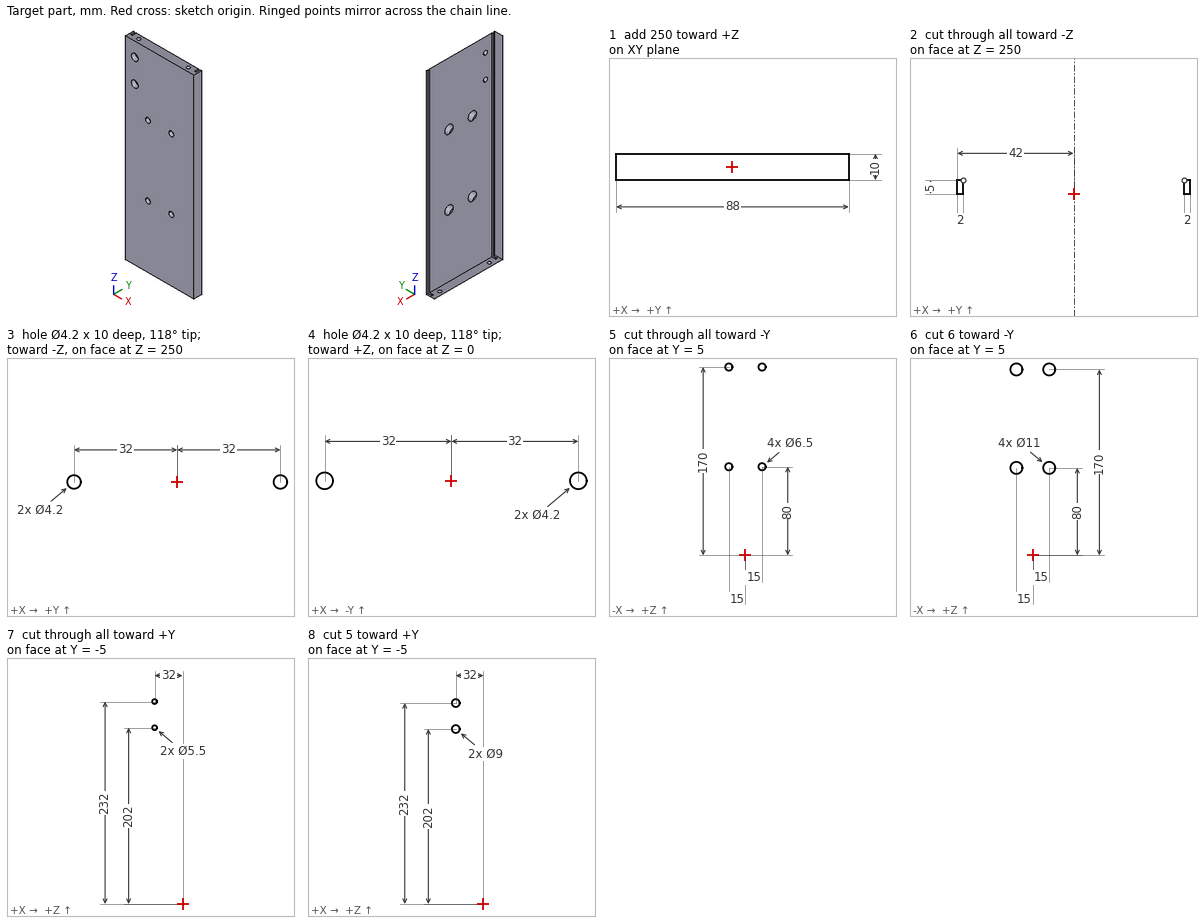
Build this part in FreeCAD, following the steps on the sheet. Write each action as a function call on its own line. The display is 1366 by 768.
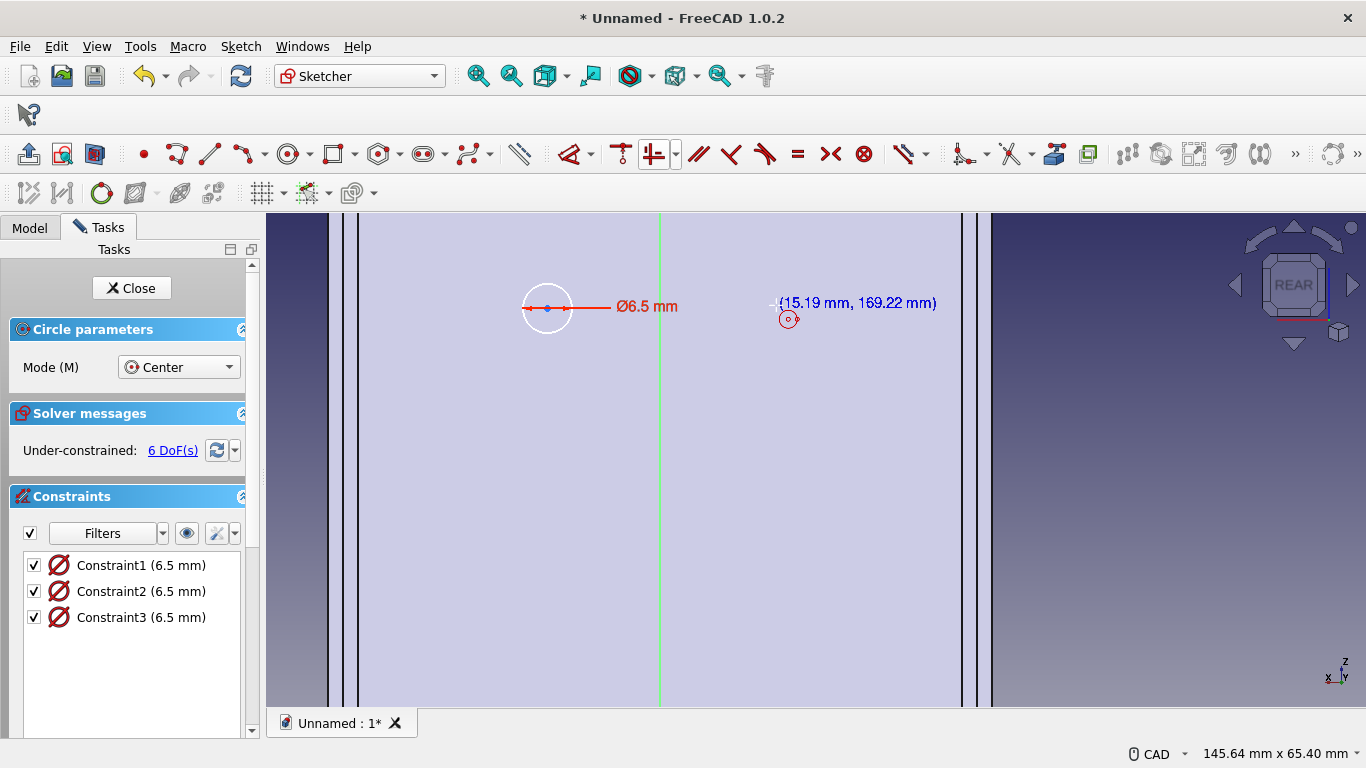
scroll(776, 305, down, 7)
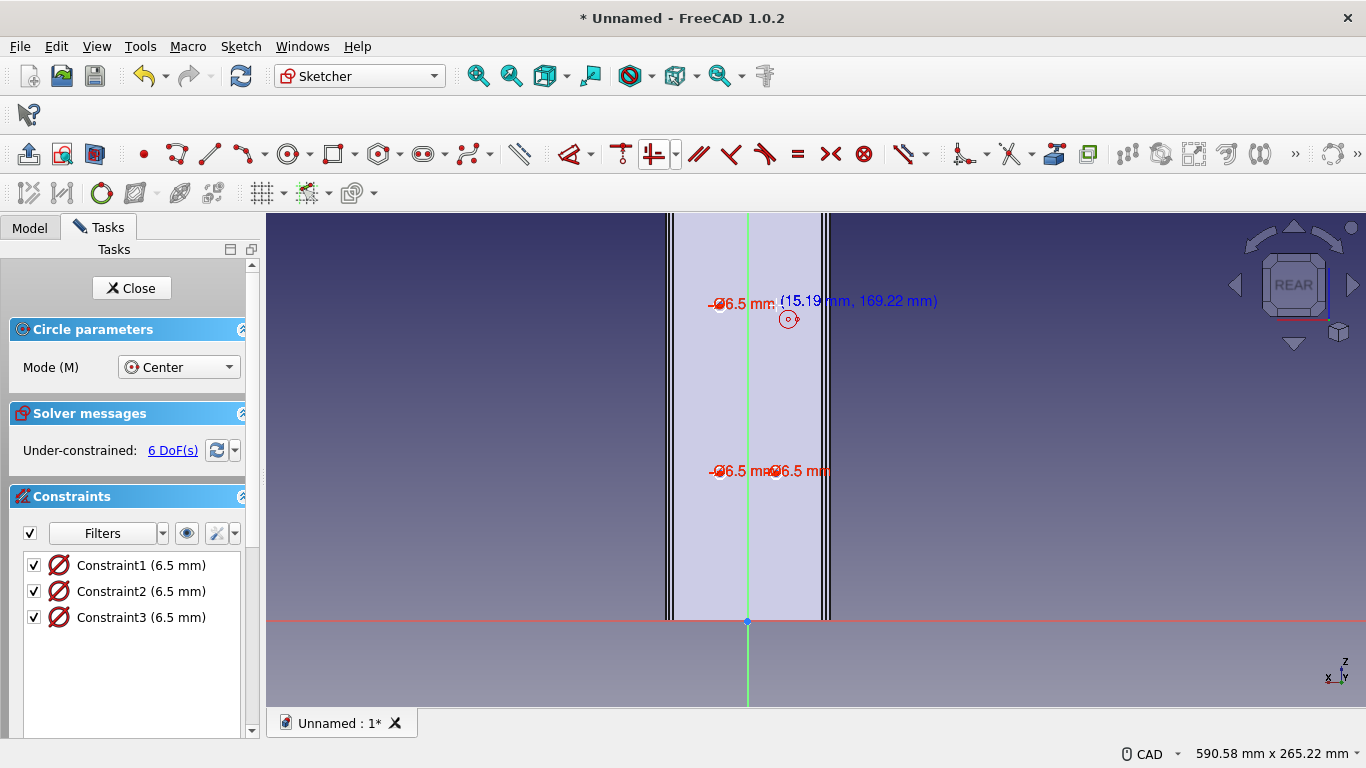
click(776, 305)
move(780, 300)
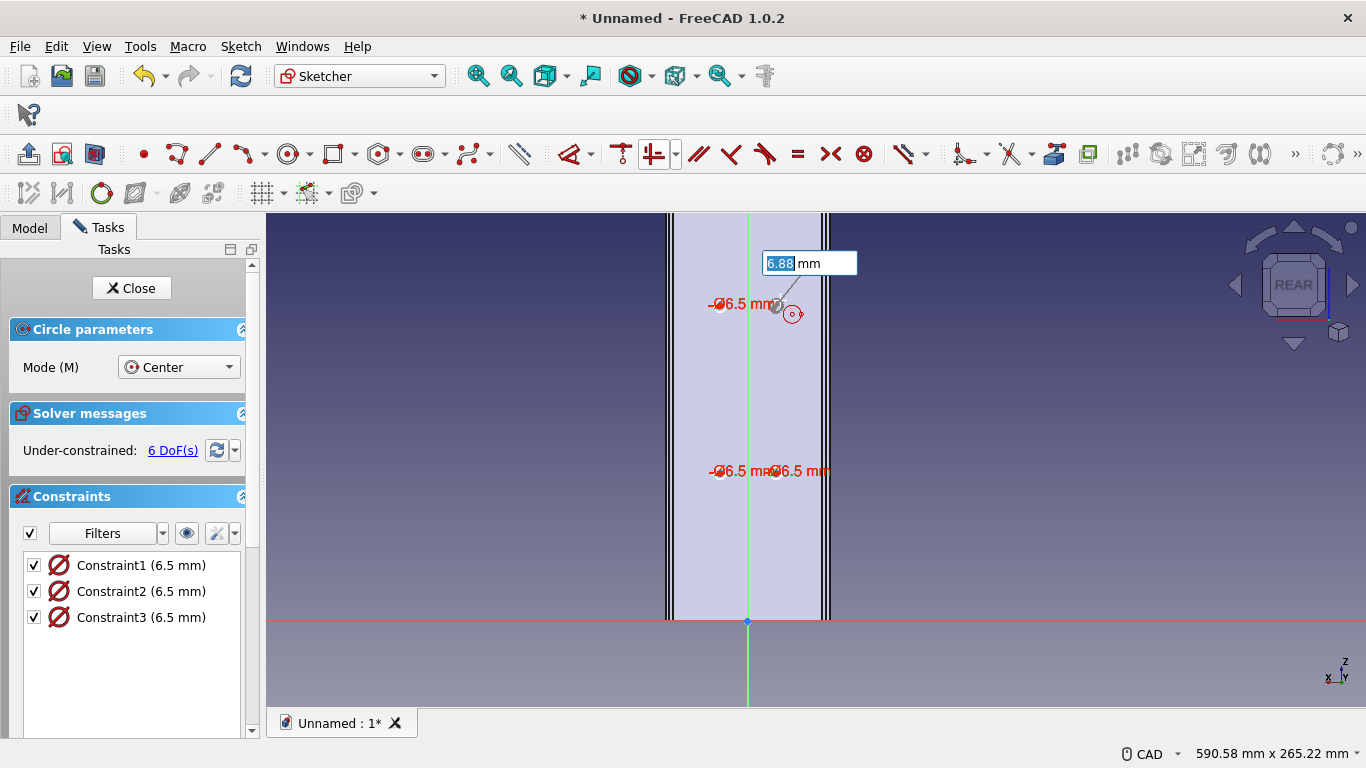
text(6.5)
key(Return)
key(Escape)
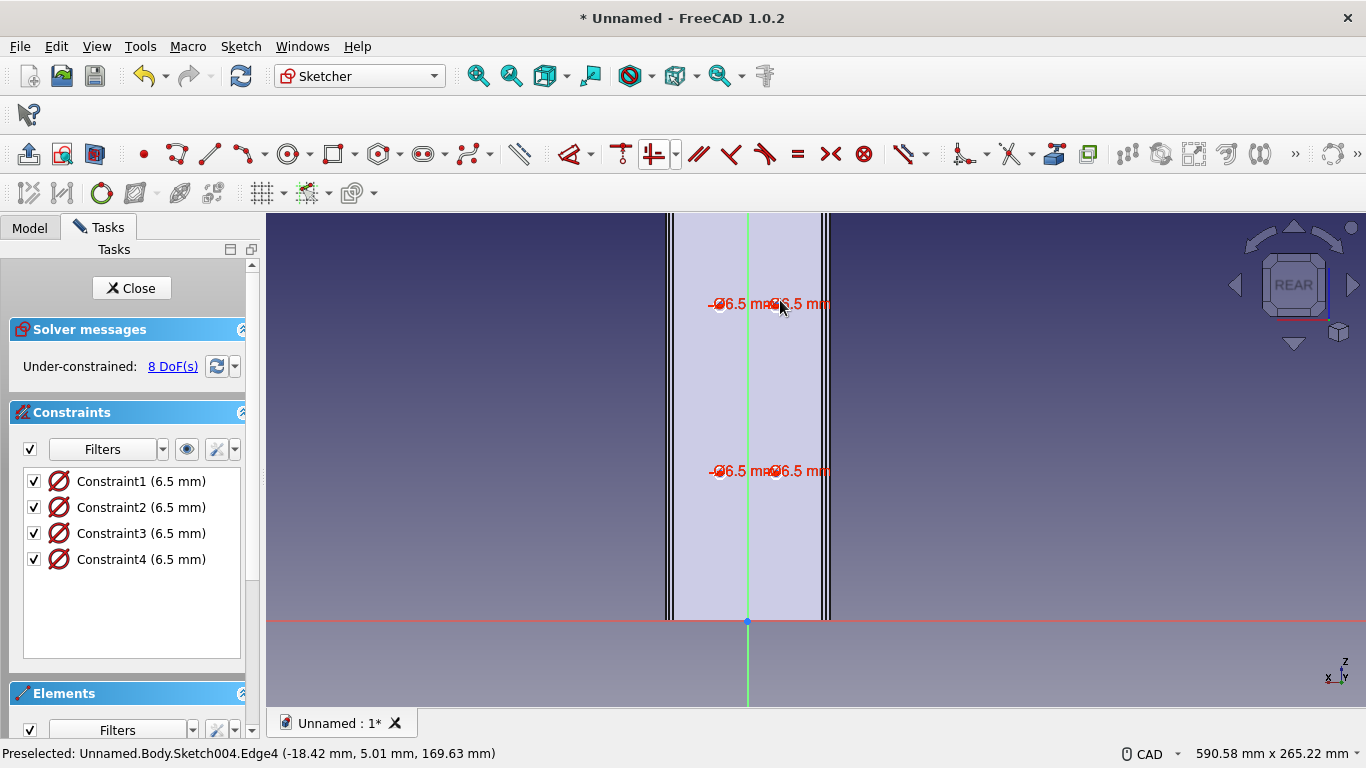
click(776, 473)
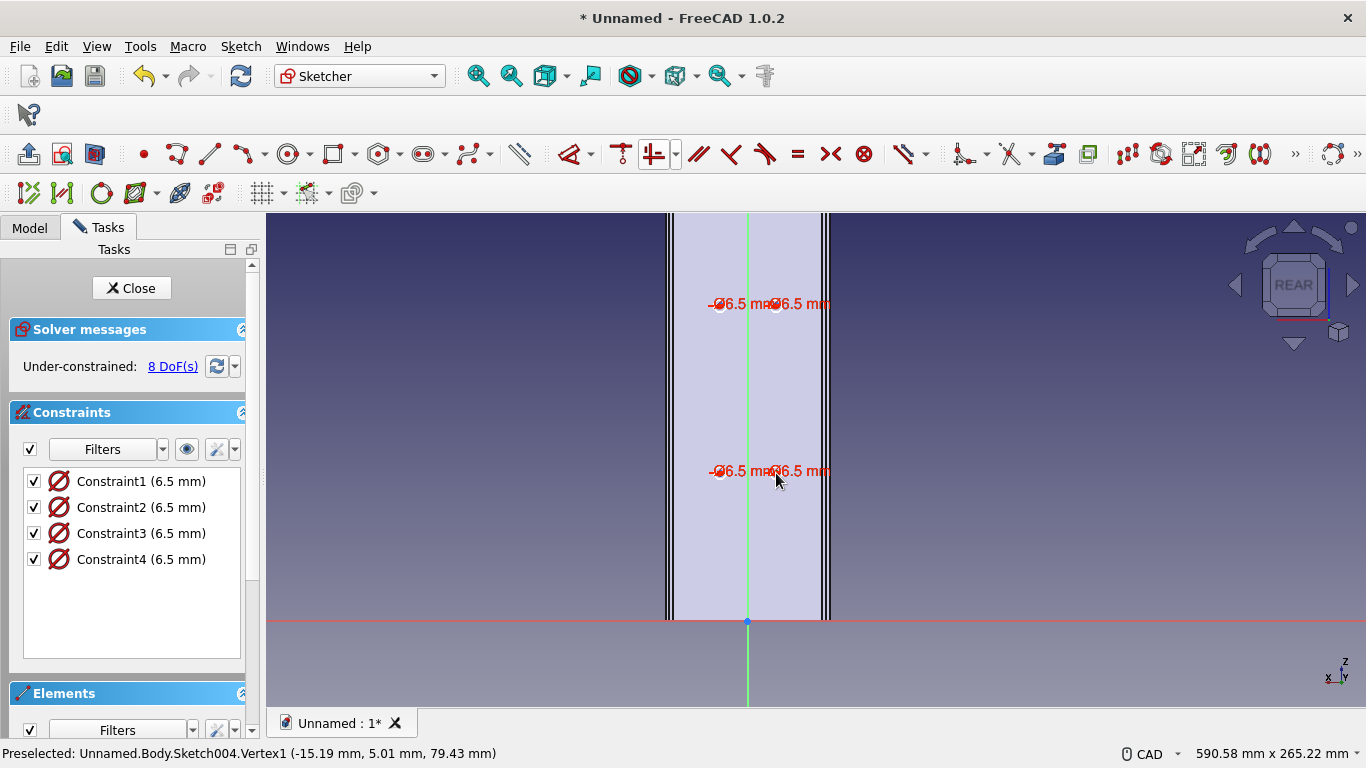
click(720, 473)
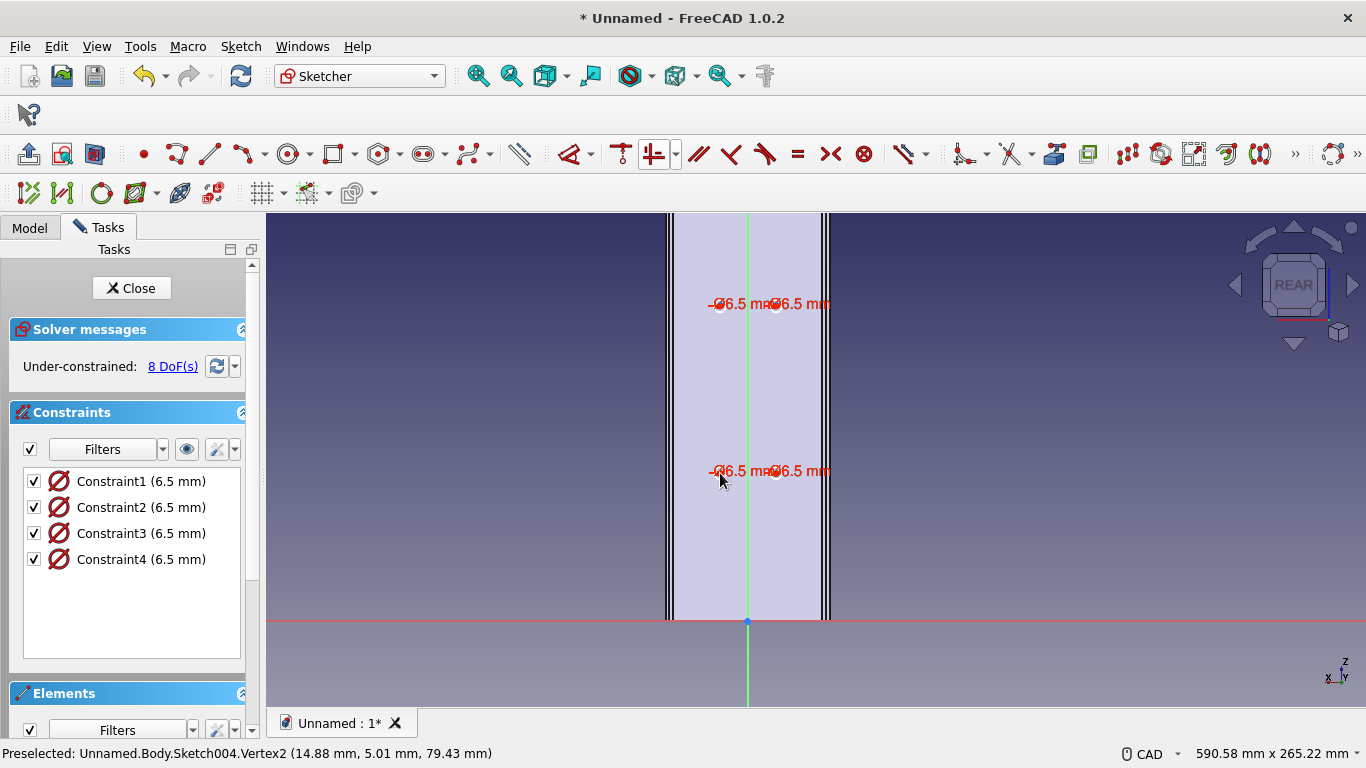
click(676, 154)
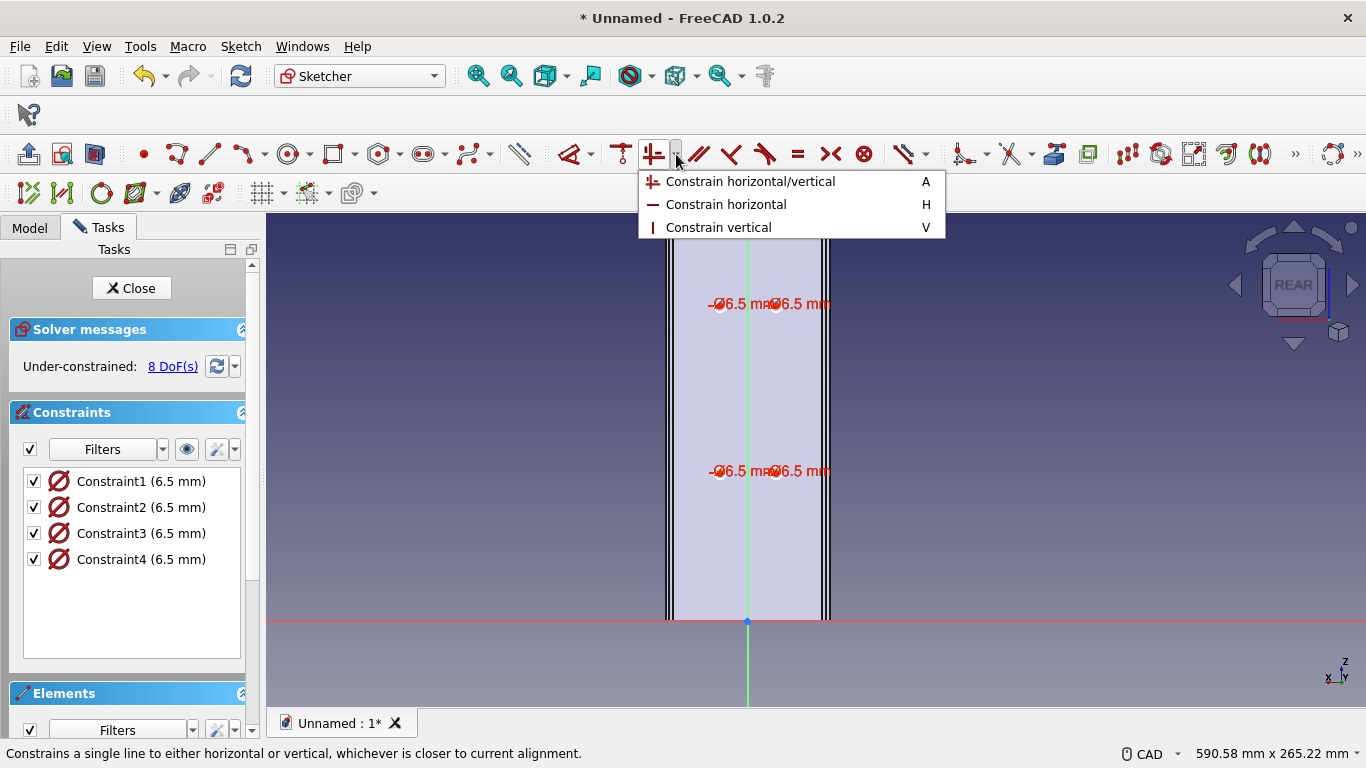
click(792, 204)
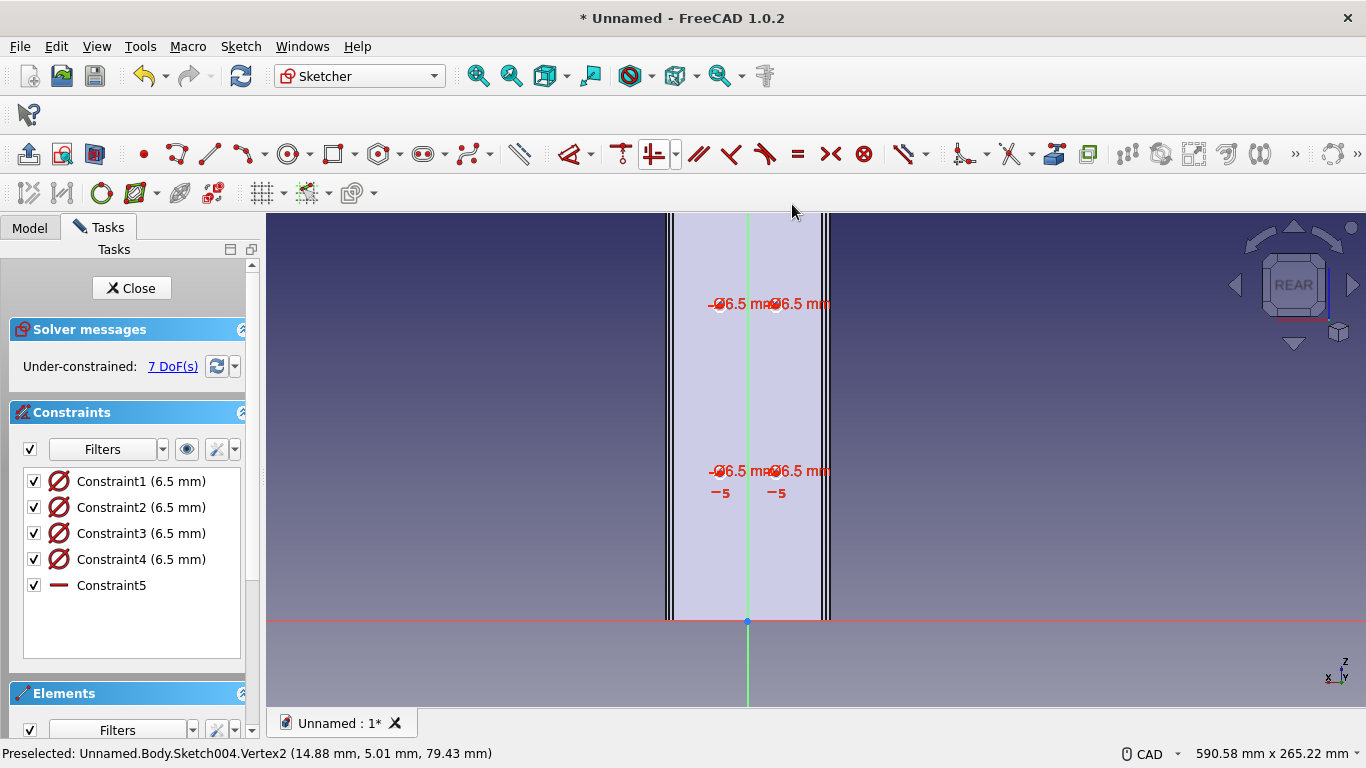
click(720, 473)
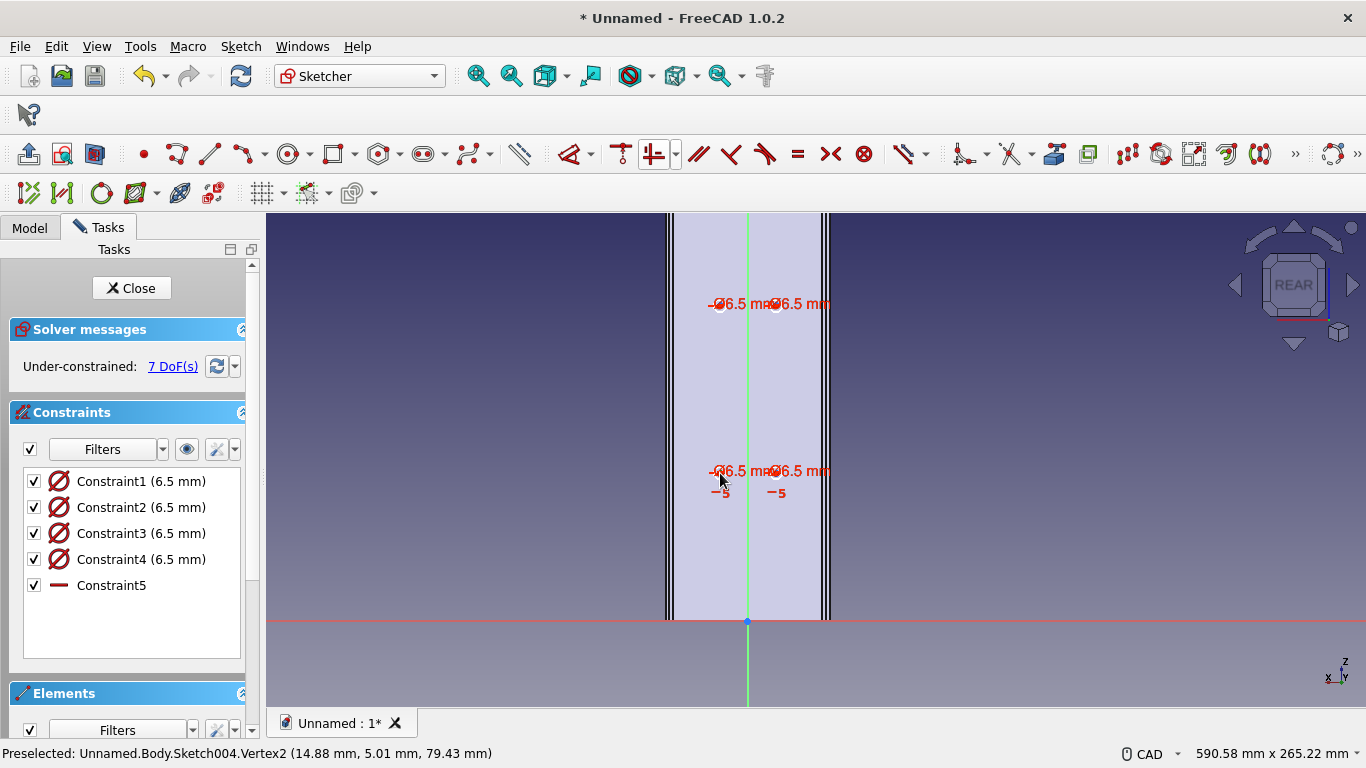
click(720, 306)